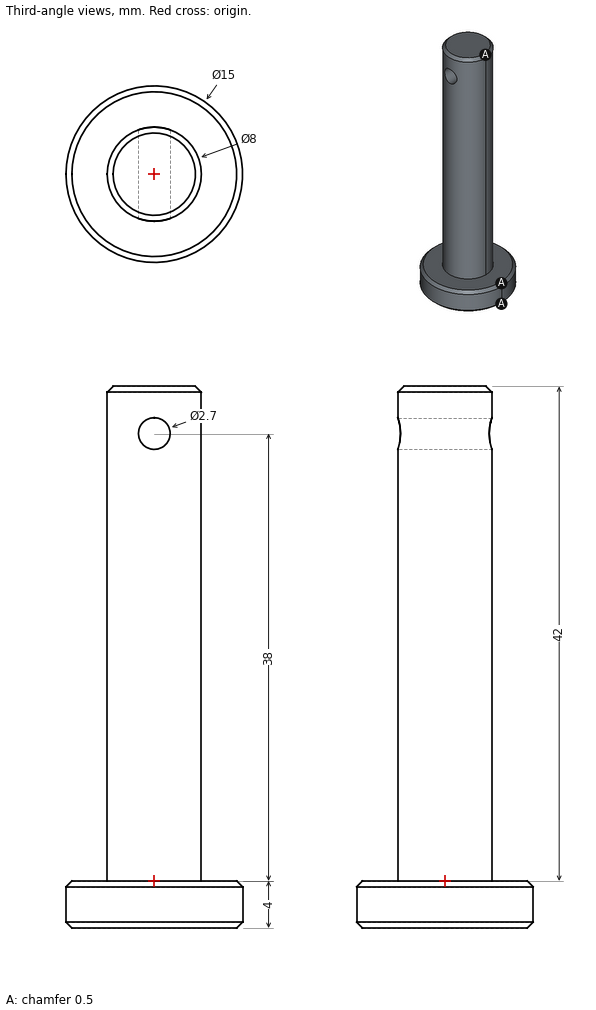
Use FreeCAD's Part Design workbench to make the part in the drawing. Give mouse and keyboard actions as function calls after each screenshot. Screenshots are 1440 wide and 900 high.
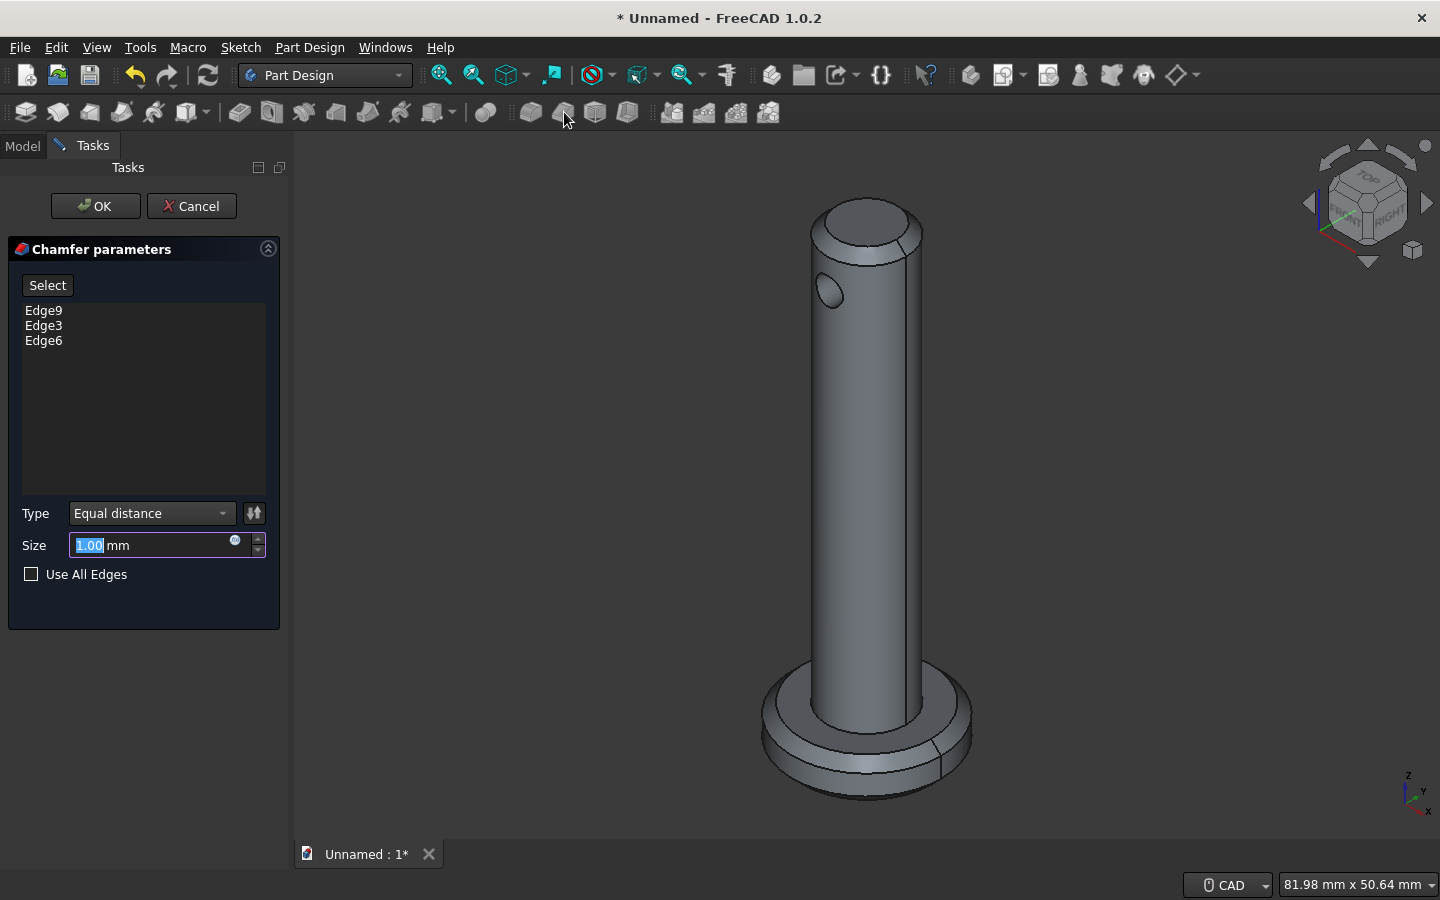
text(0.5)
key(Tab)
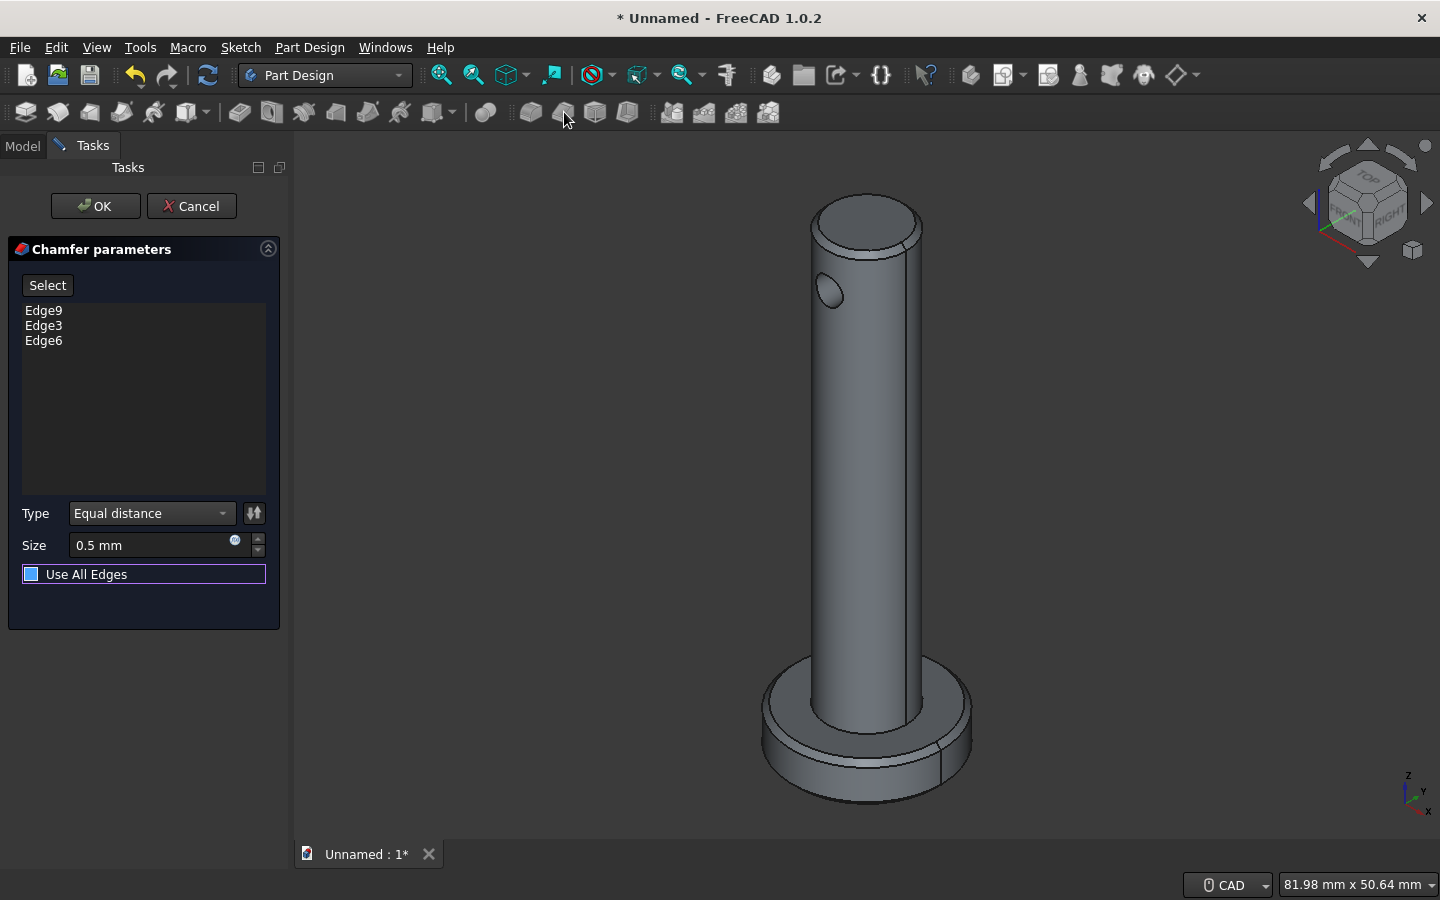
click(96, 206)